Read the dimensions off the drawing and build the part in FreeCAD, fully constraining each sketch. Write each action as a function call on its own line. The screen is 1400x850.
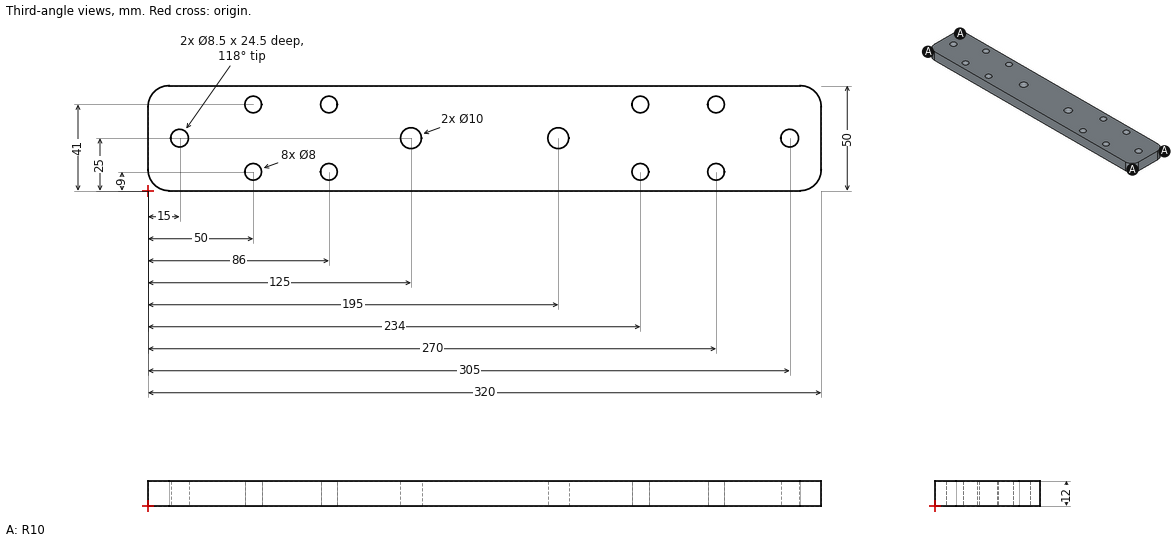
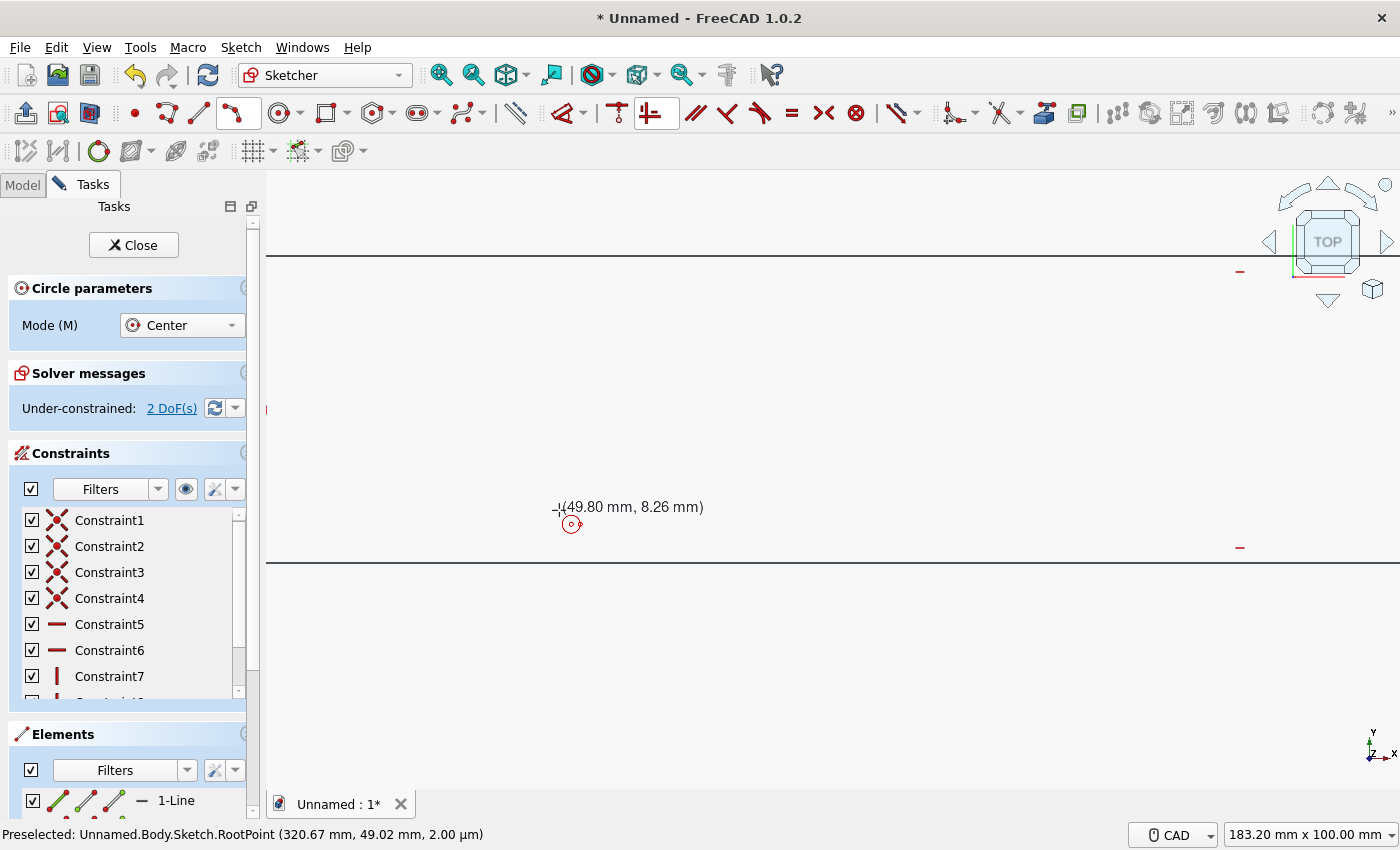
click(560, 507)
click(577, 490)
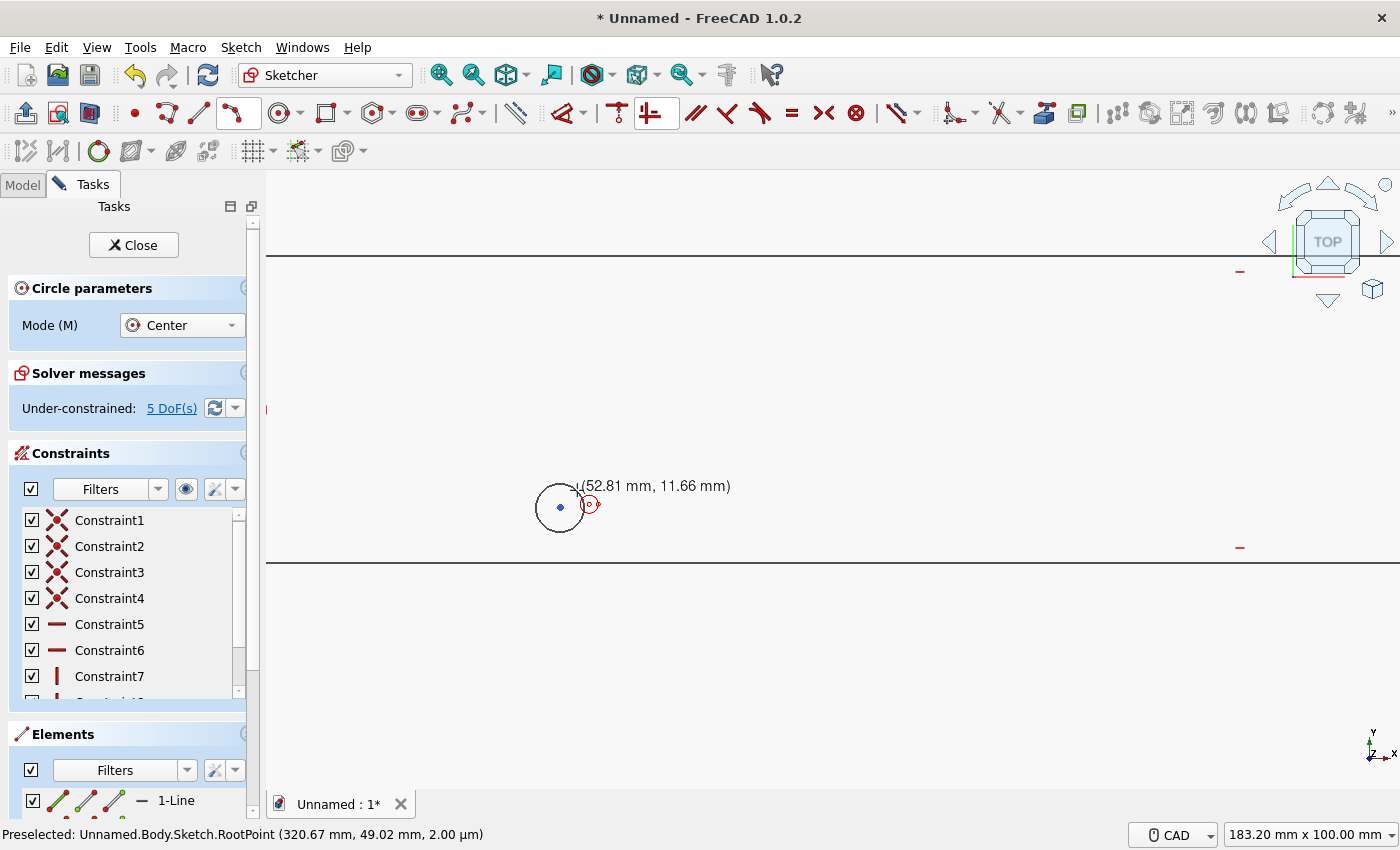
click(782, 507)
click(800, 490)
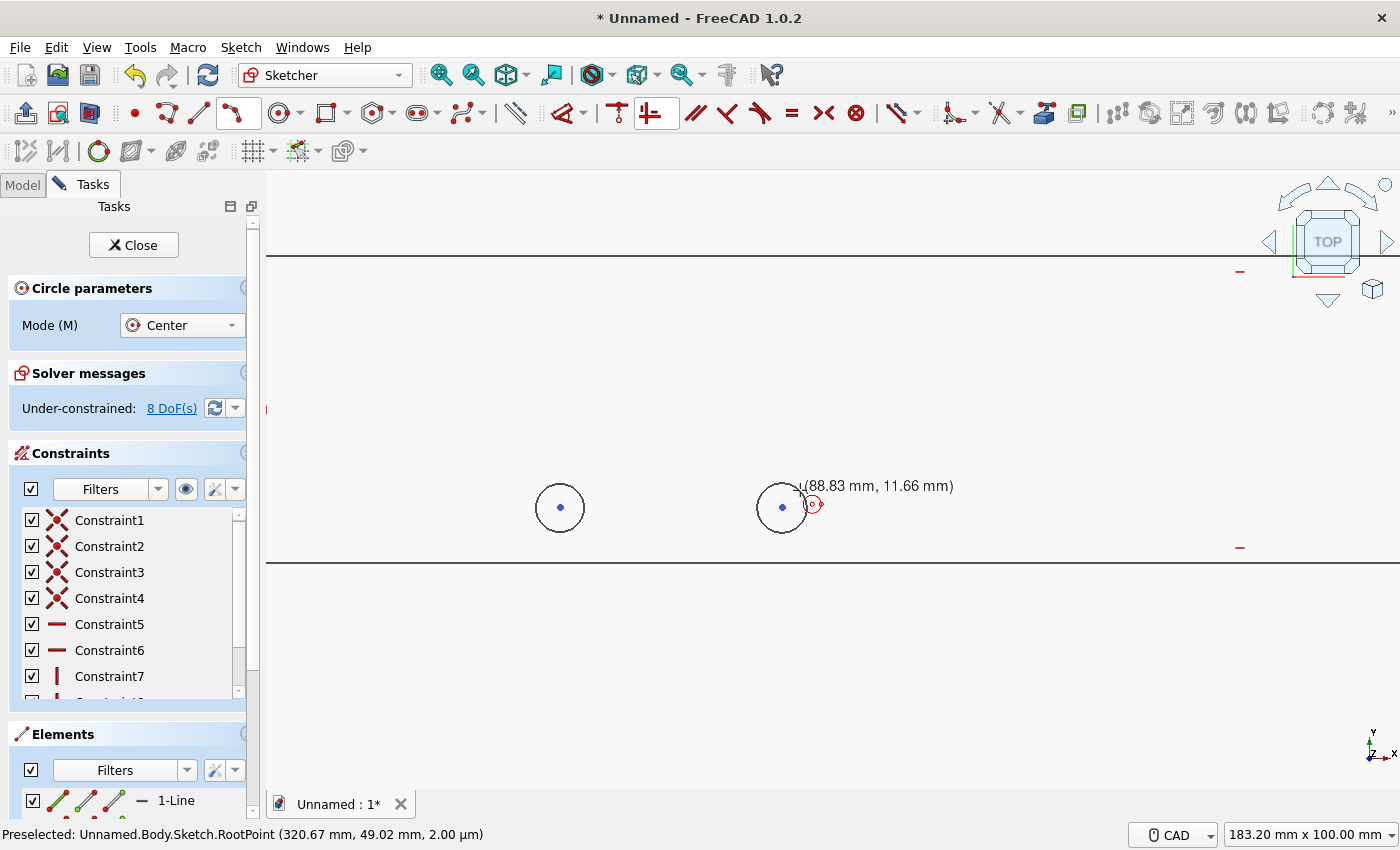
scroll(487, 521, down, 5)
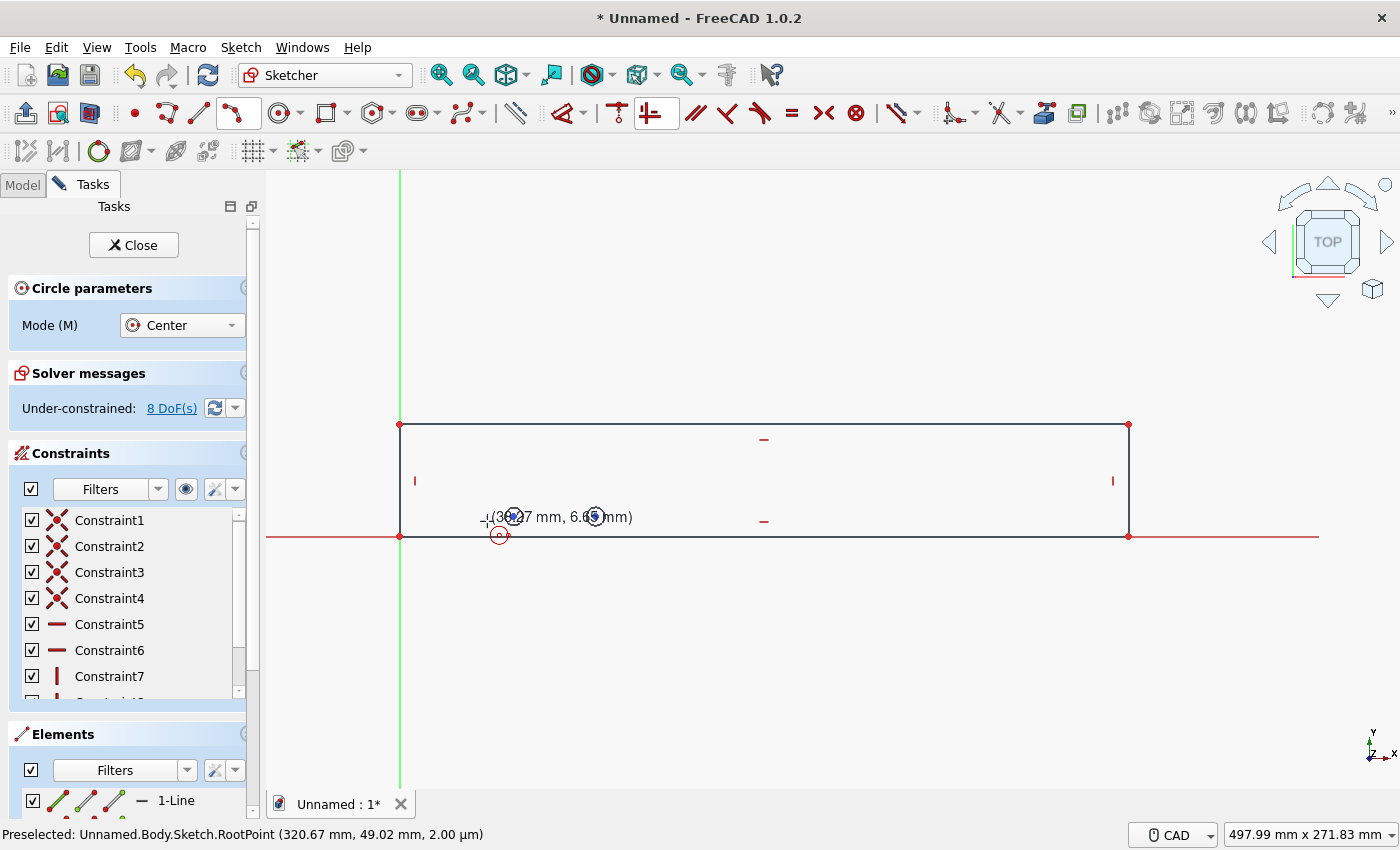
scroll(933, 516, up, 5)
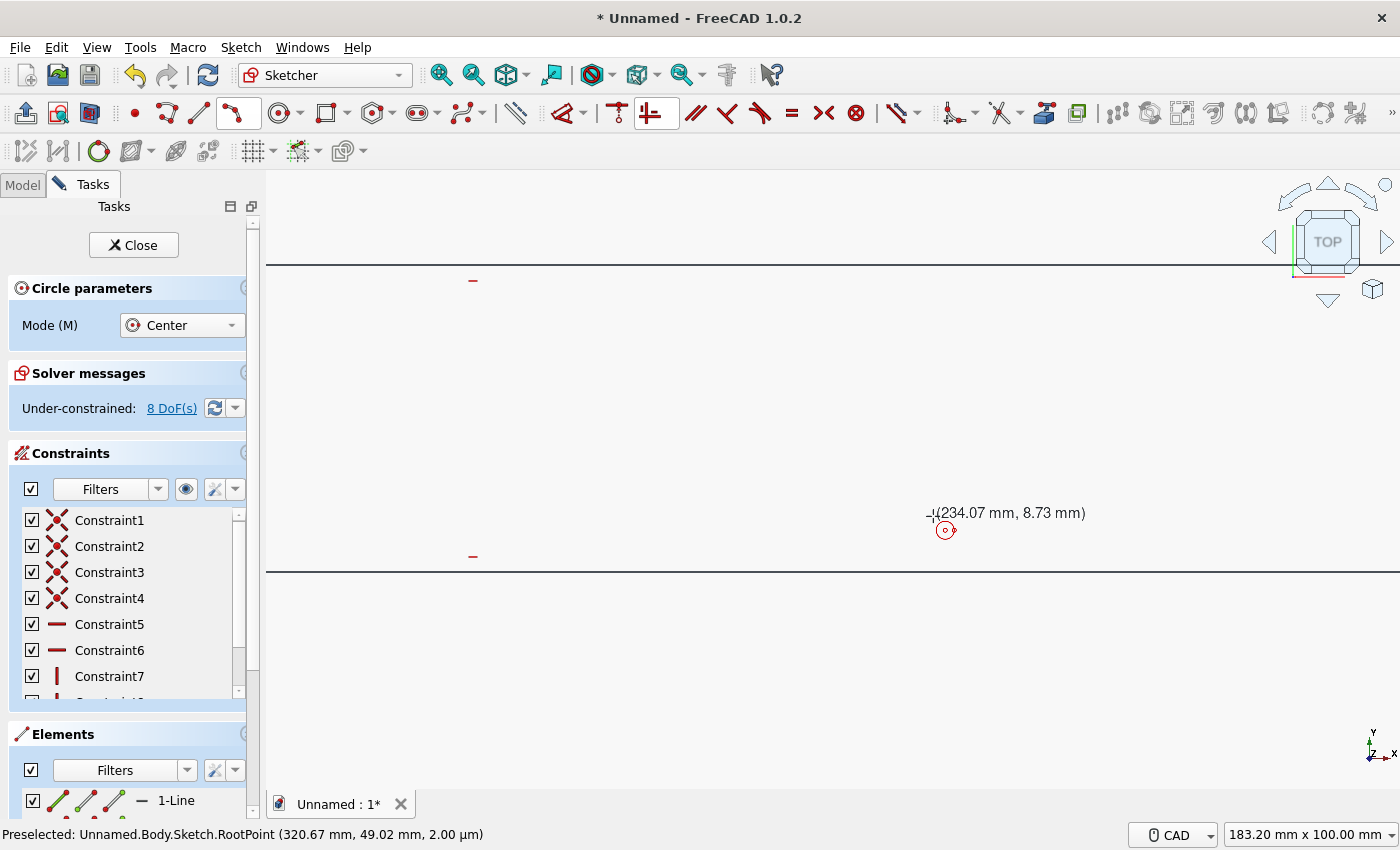
click(932, 516)
click(949, 499)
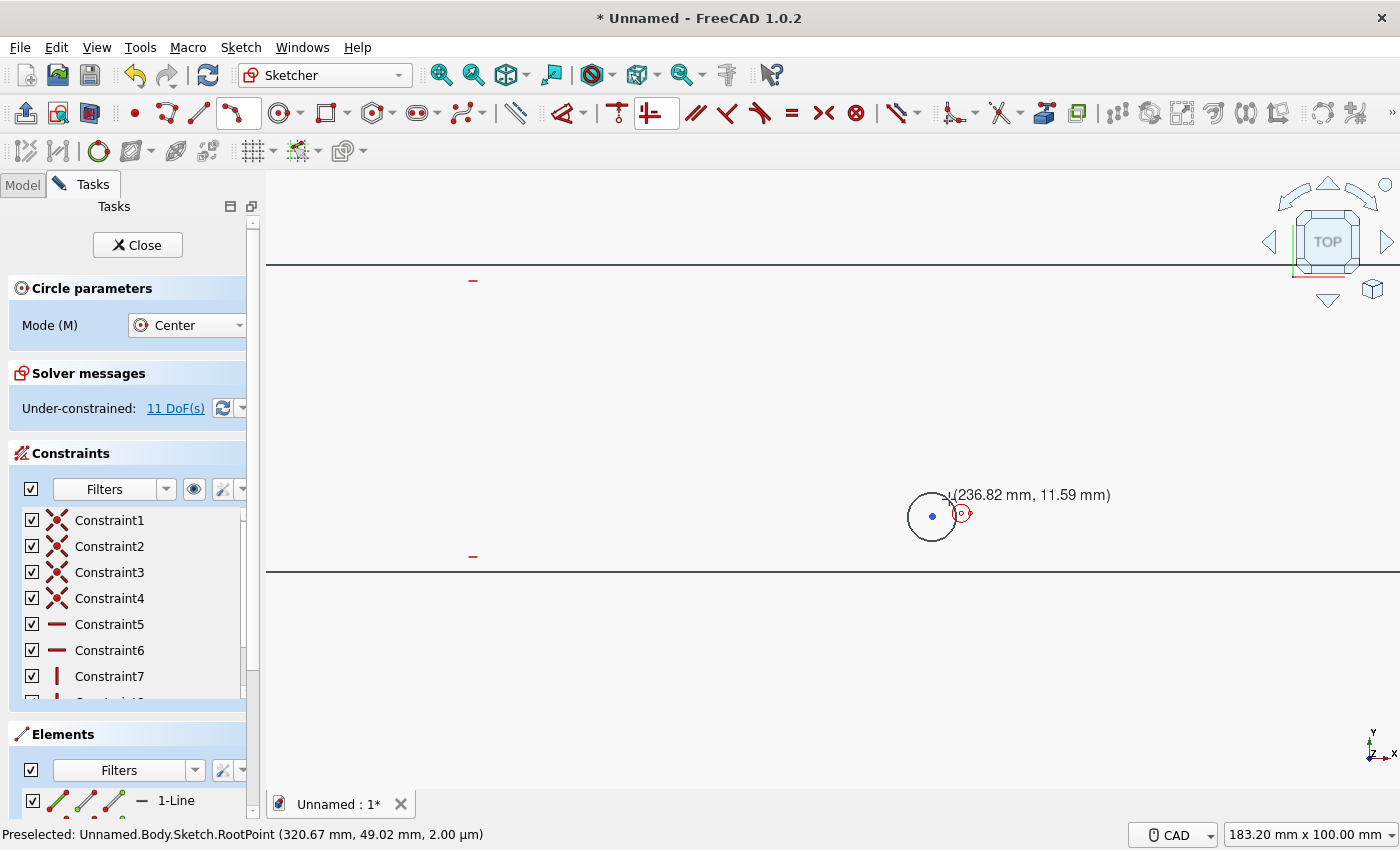
click(1154, 516)
click(1172, 499)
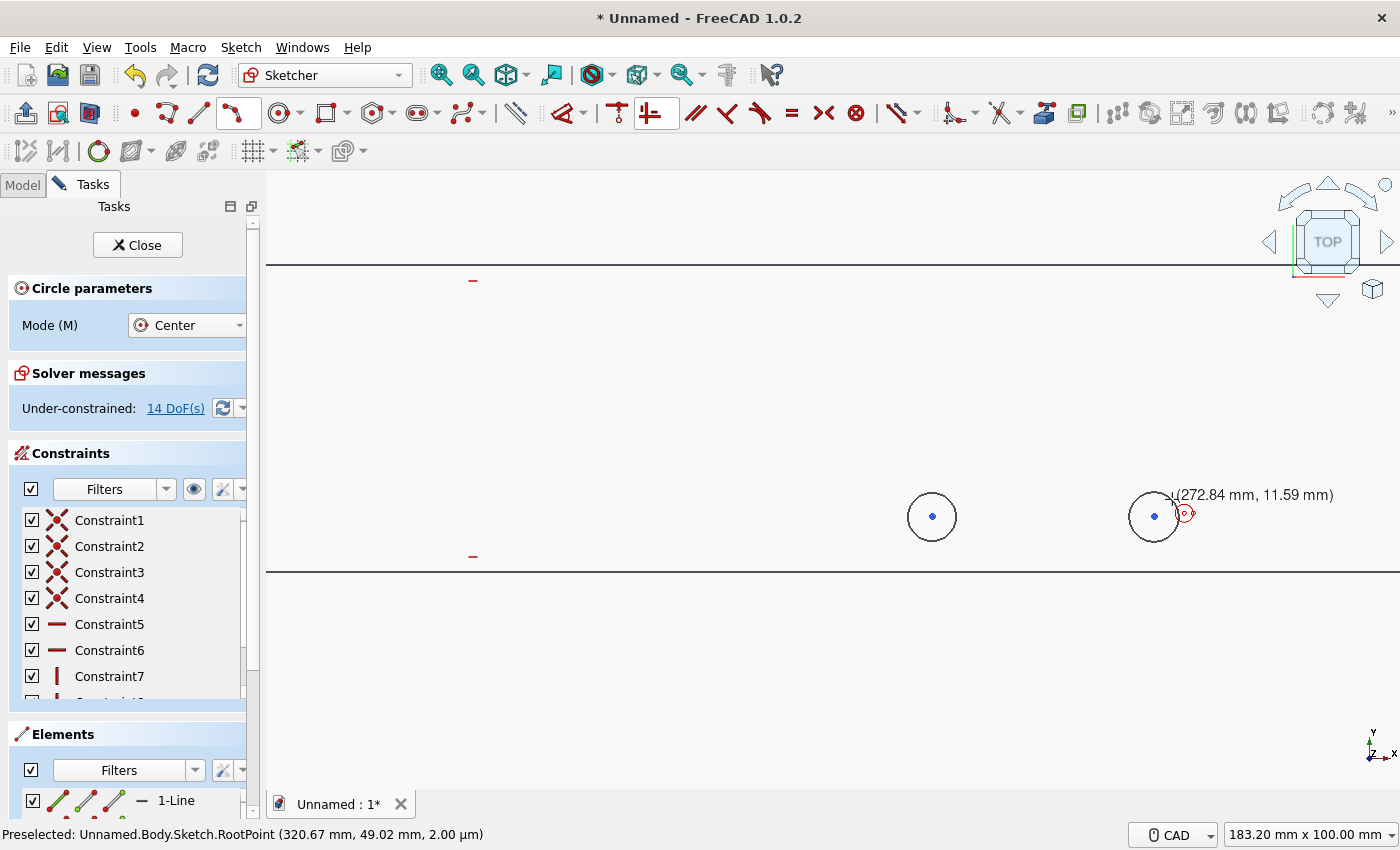
scroll(934, 516, down, 5)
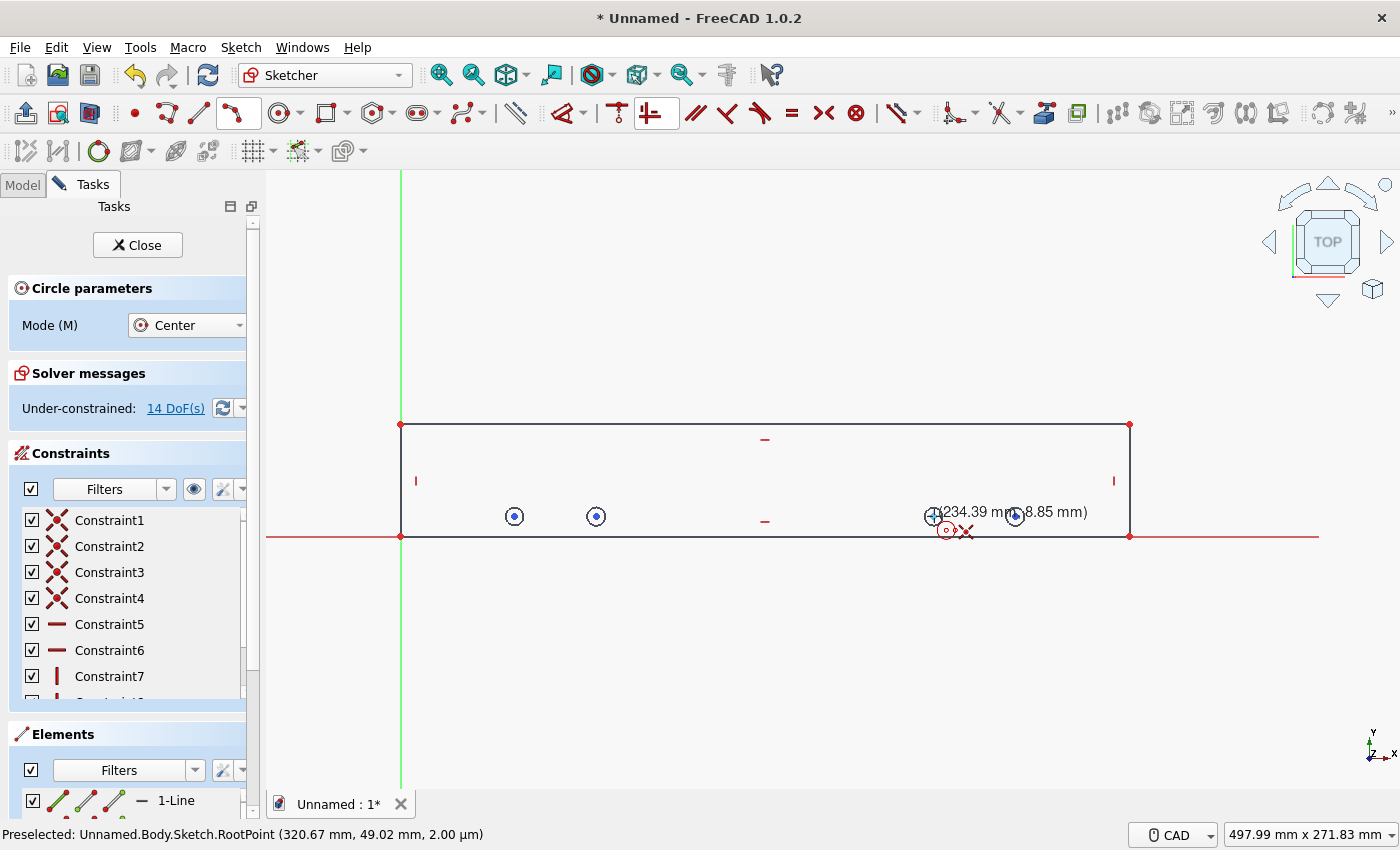
scroll(685, 480, up, 4)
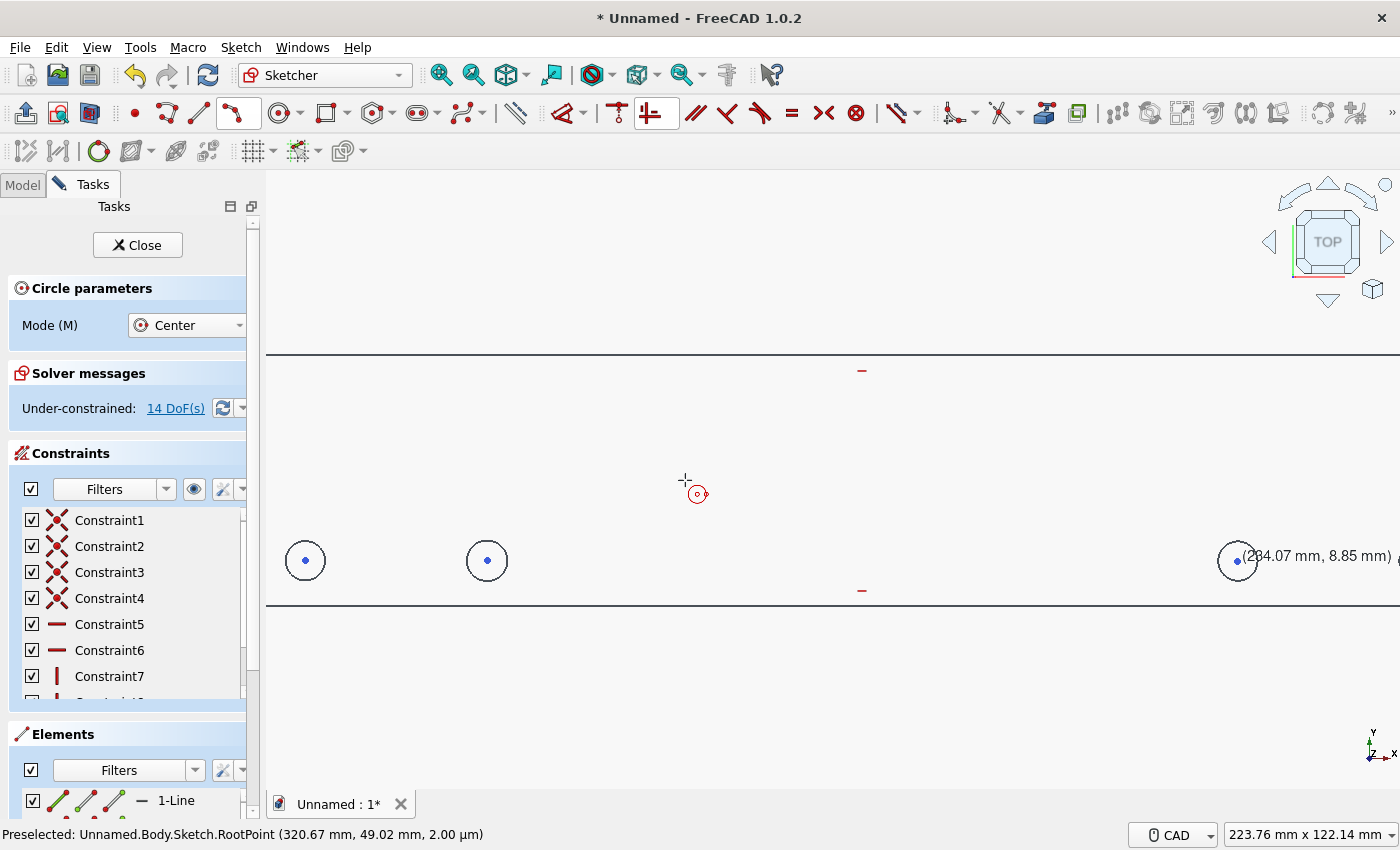
click(685, 479)
click(703, 461)